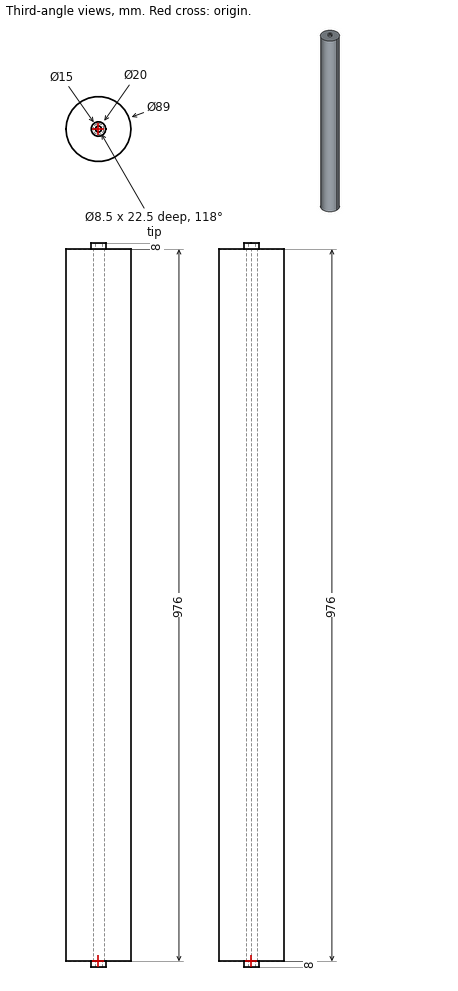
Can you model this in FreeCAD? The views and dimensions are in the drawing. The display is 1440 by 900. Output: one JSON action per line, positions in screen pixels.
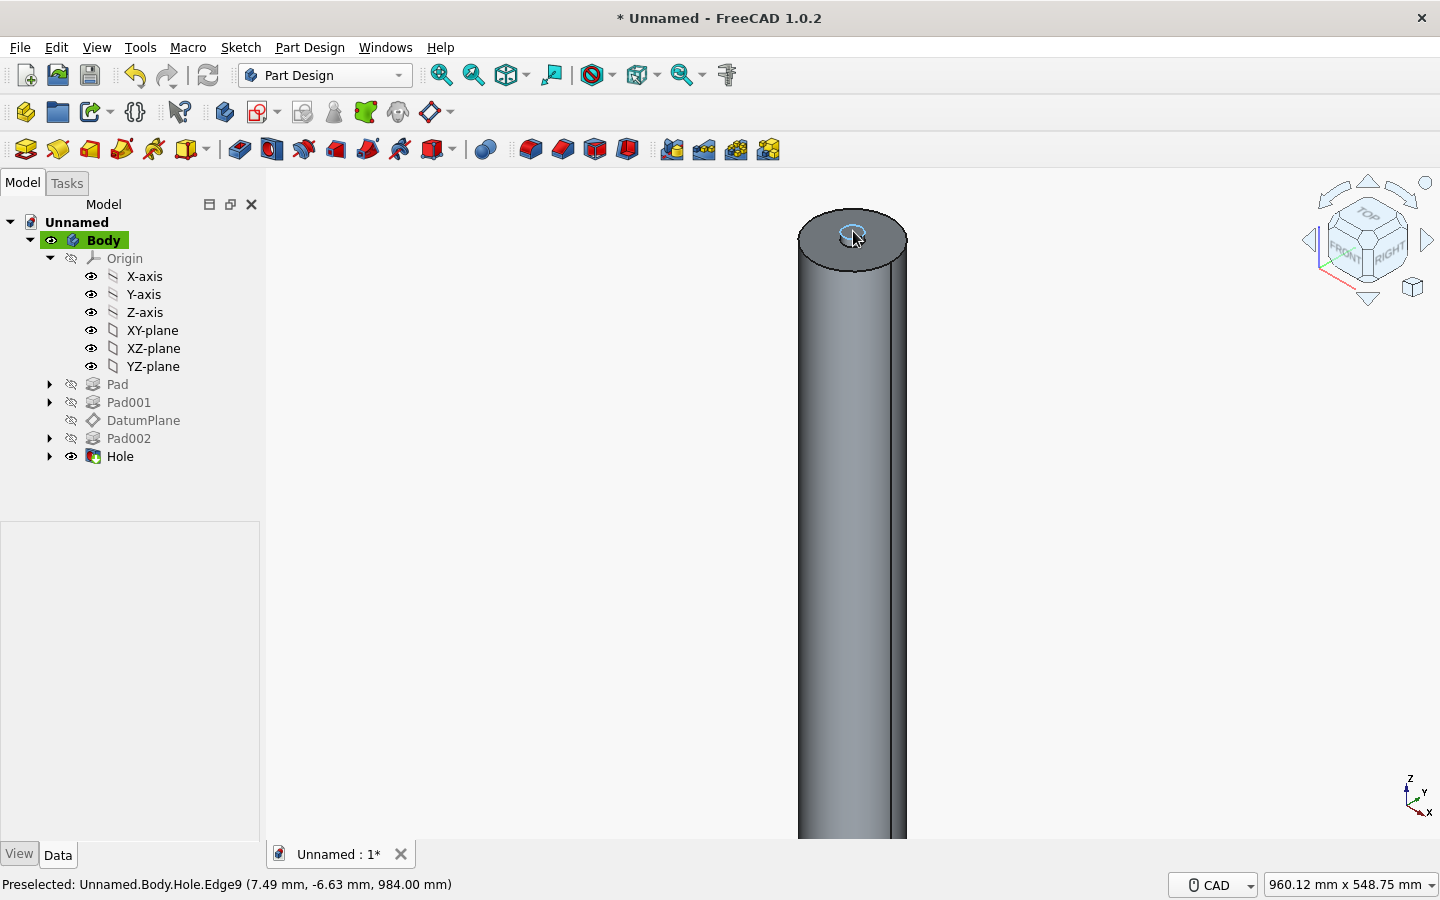
{"action": "left_click", "coordinate": [442, 76]}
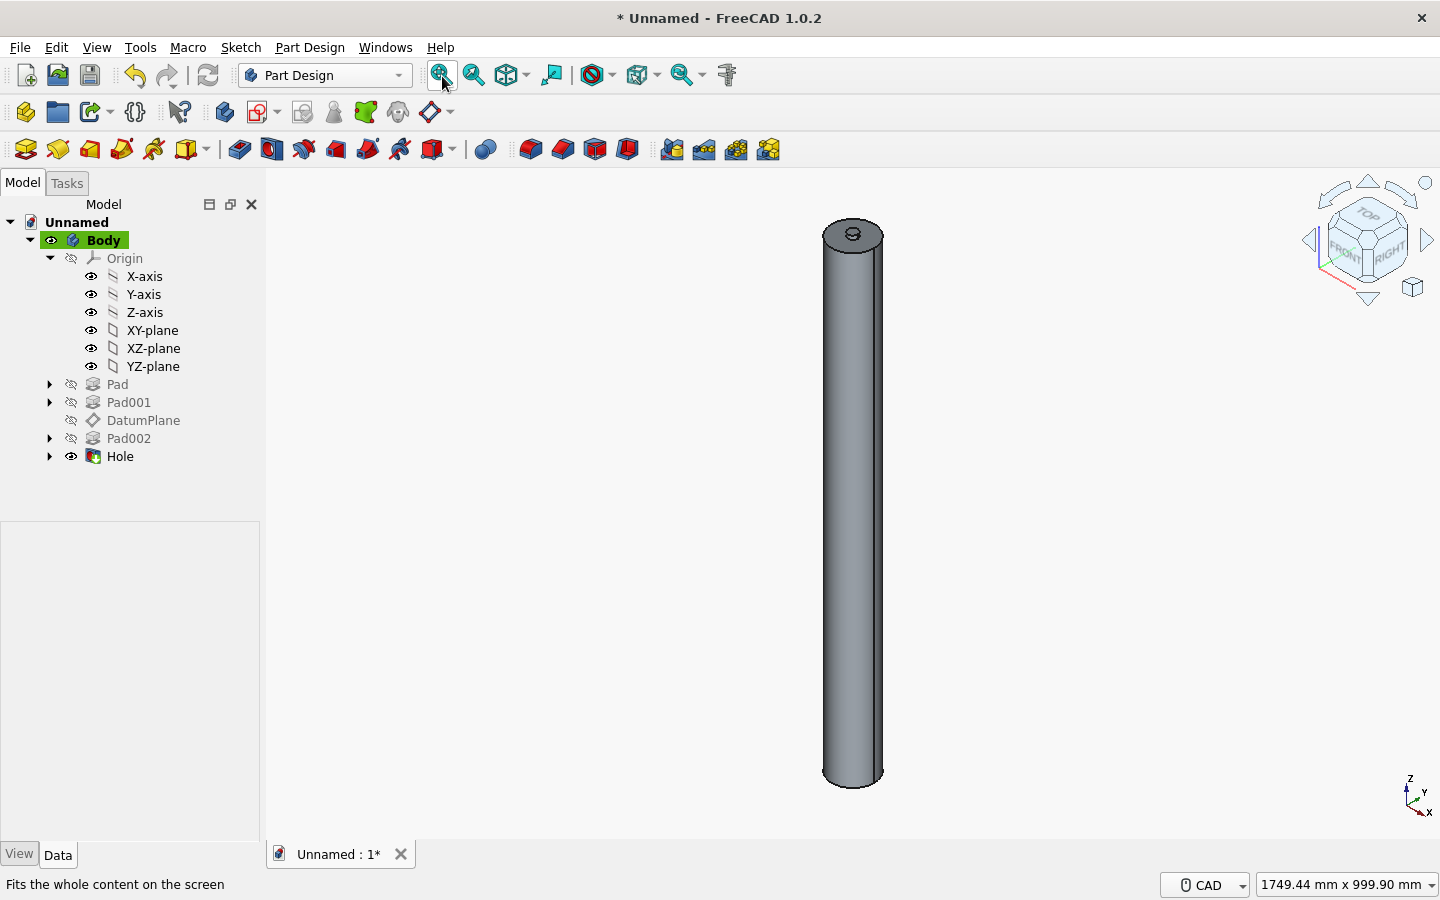
{"action": "key", "text": "2"}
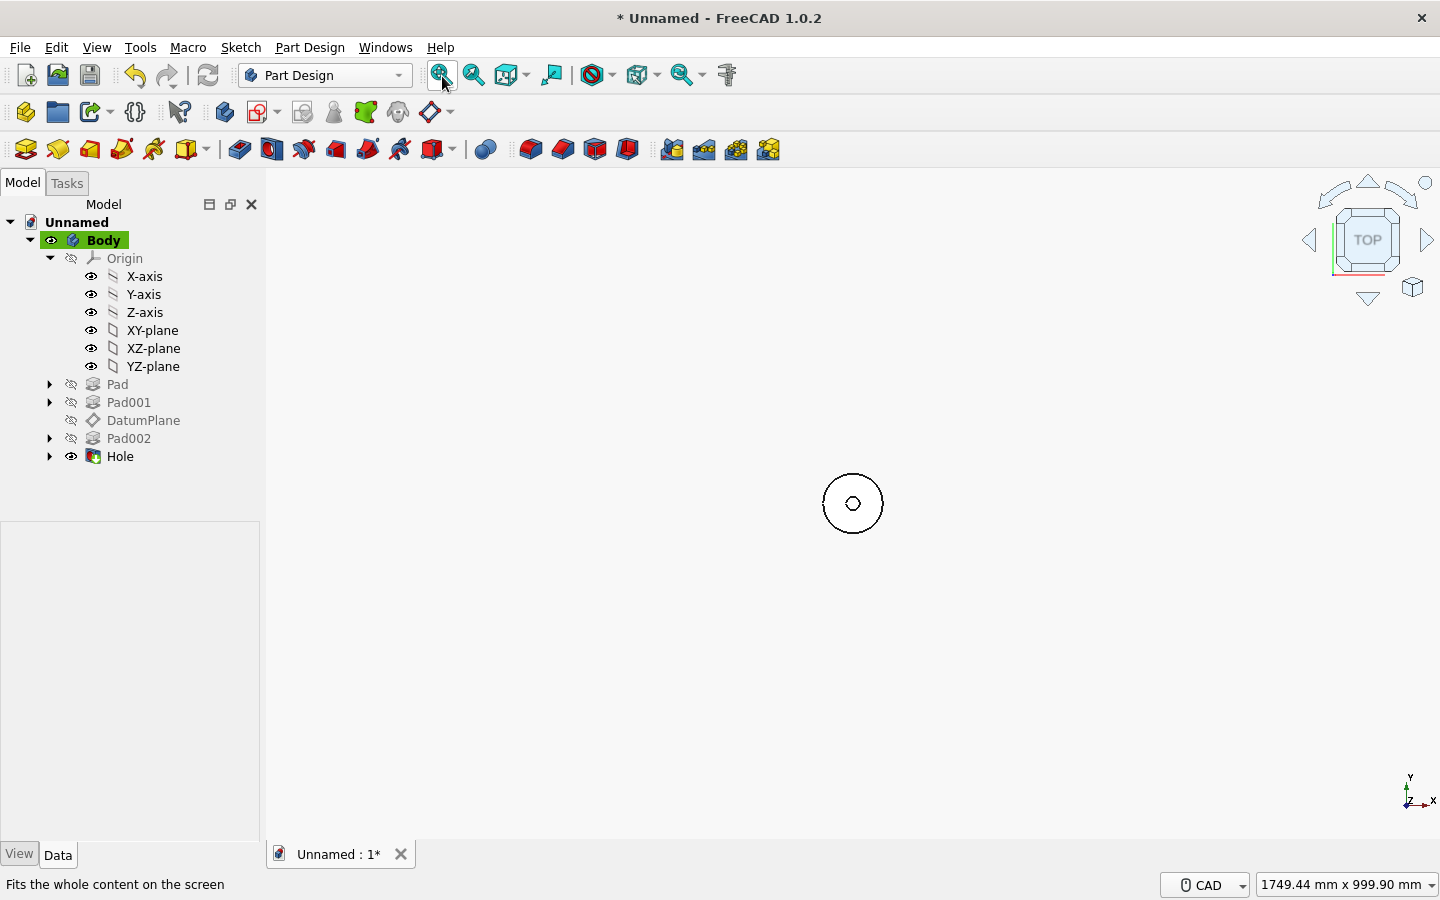
{"action": "left_click", "coordinate": [442, 76]}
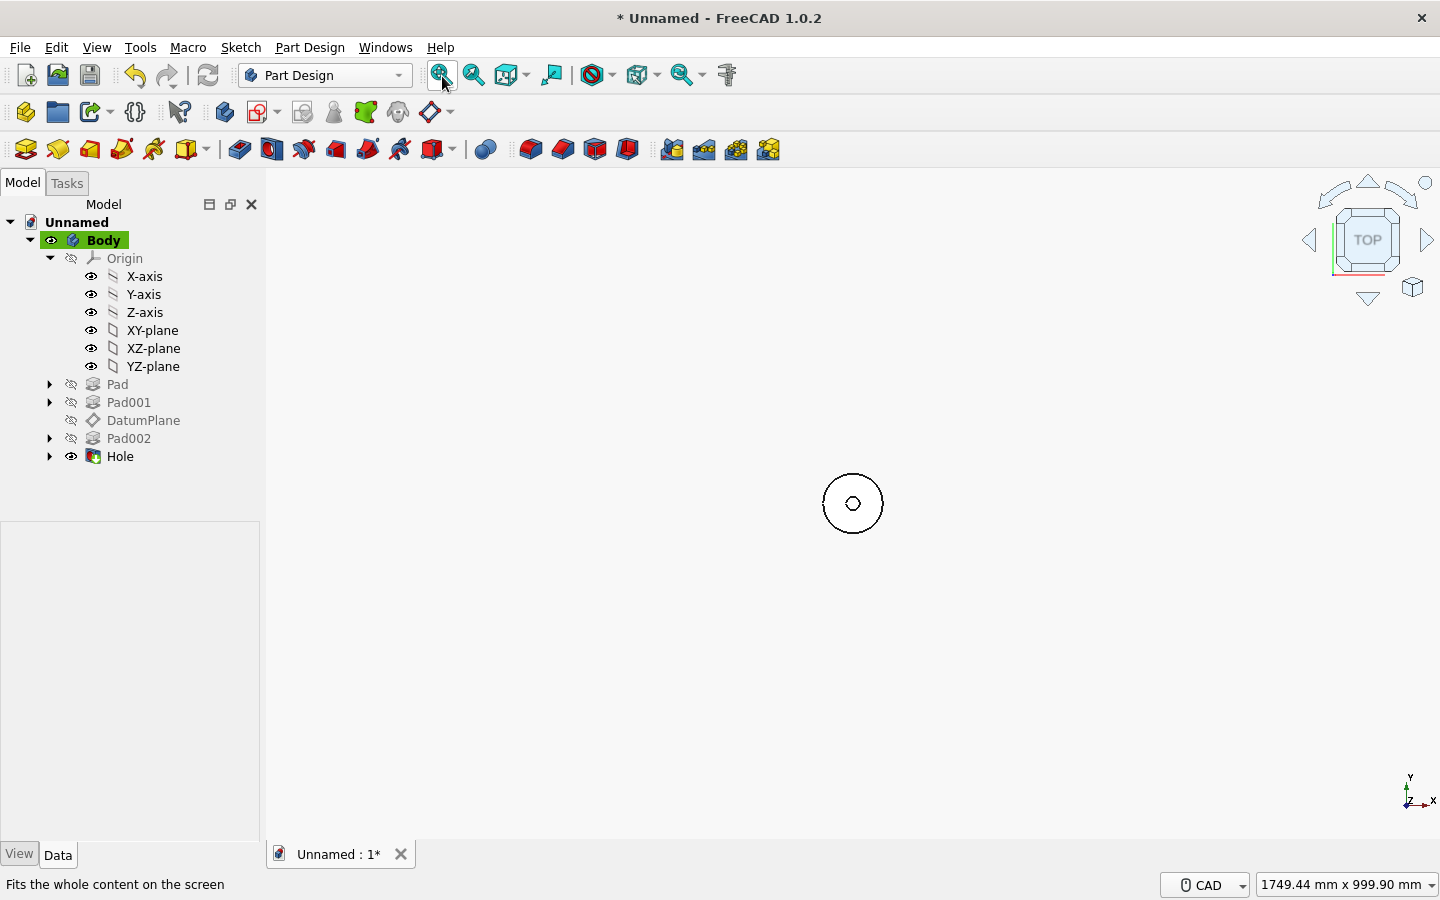
{"action": "scroll", "coordinate": [853, 502], "scroll_direction": "up", "scroll_amount": 3}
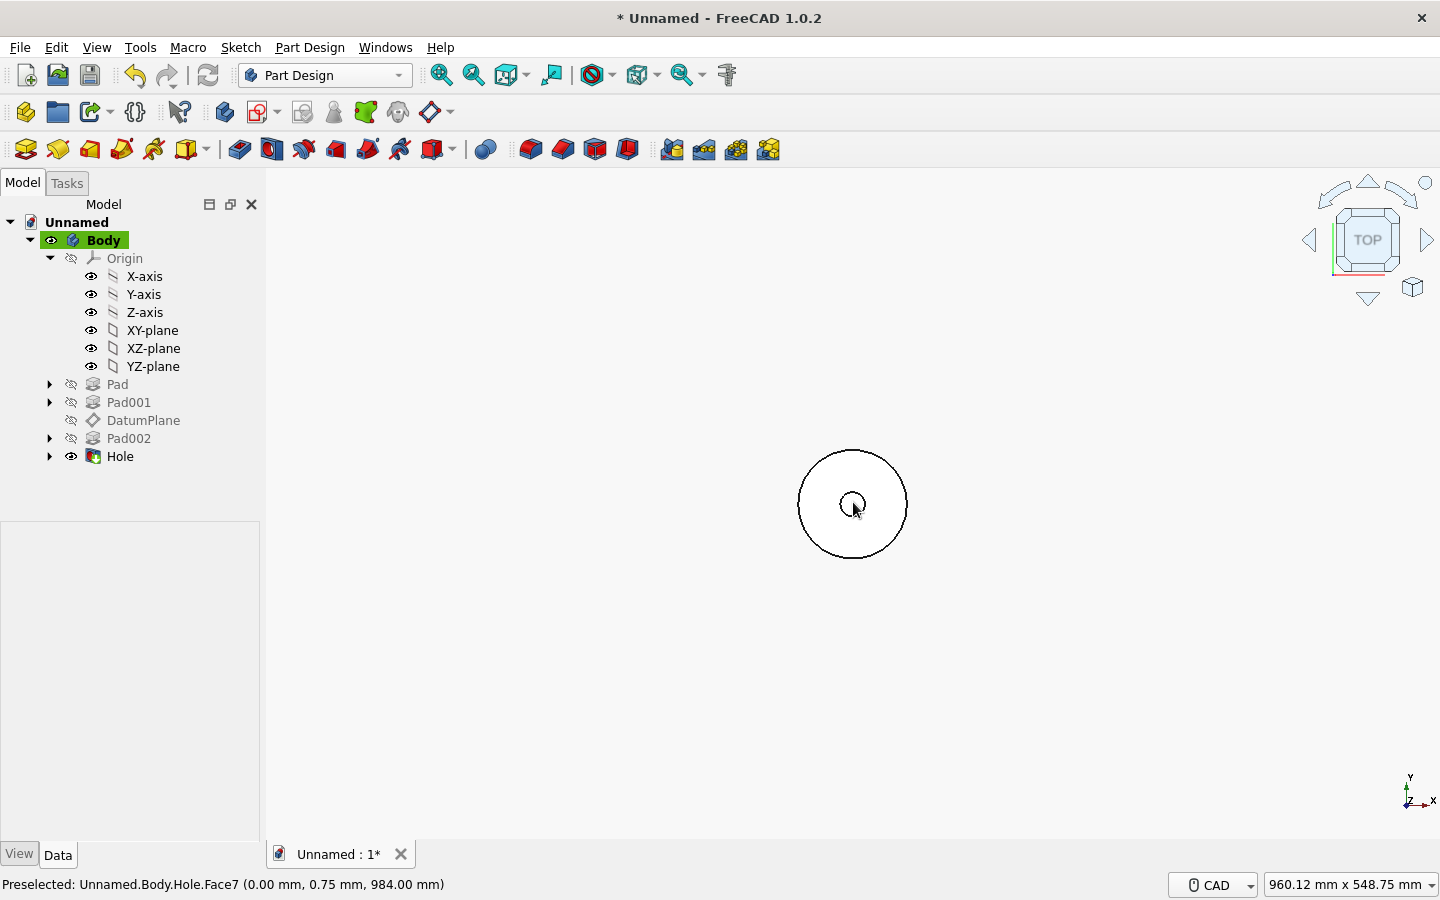
{"action": "left_click", "coordinate": [853, 503]}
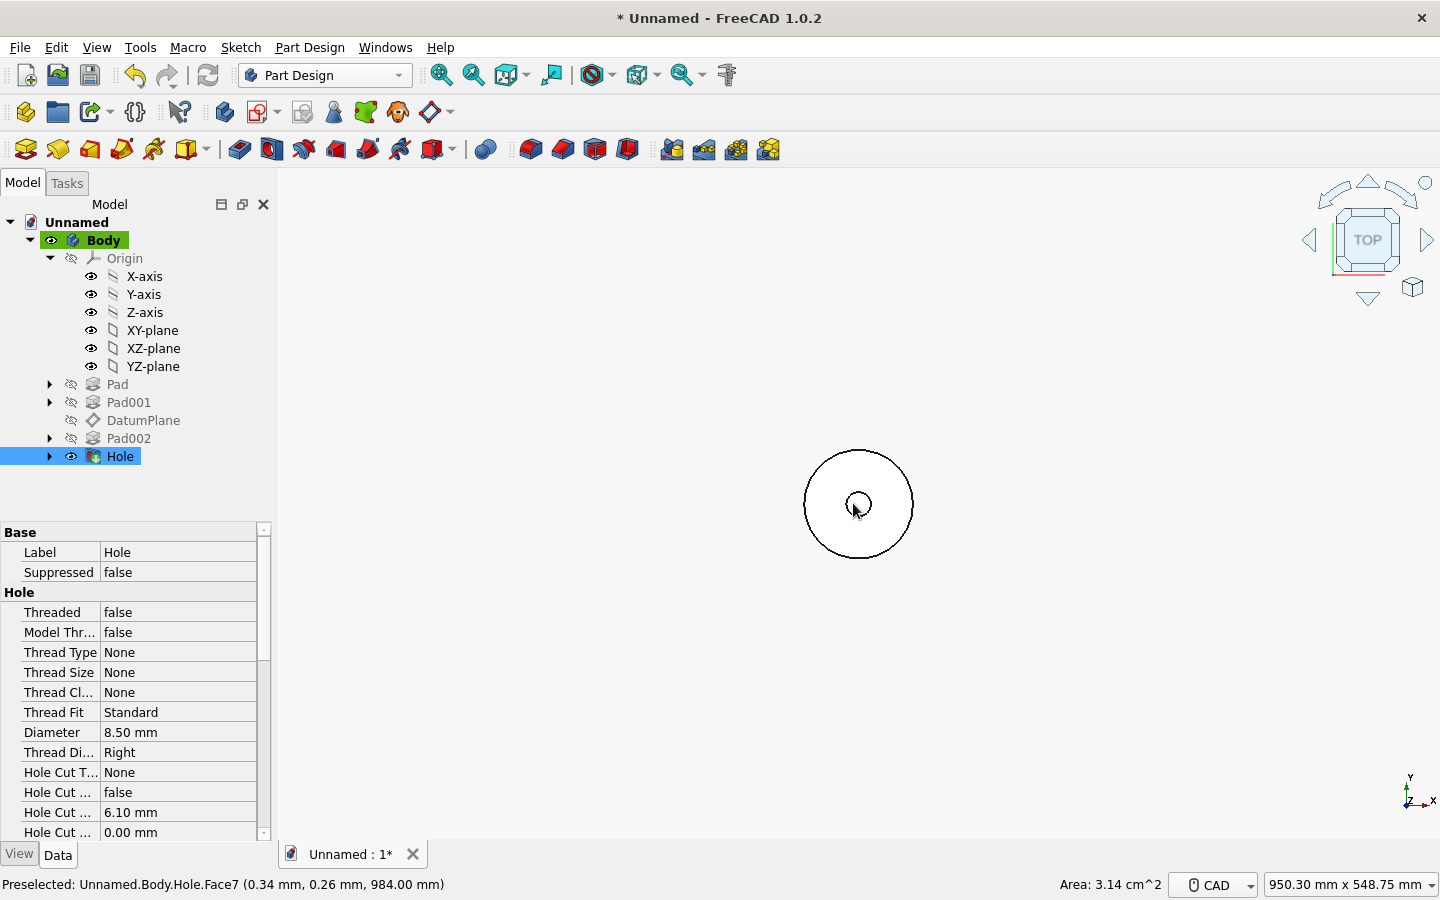
{"action": "left_click", "coordinate": [258, 112]}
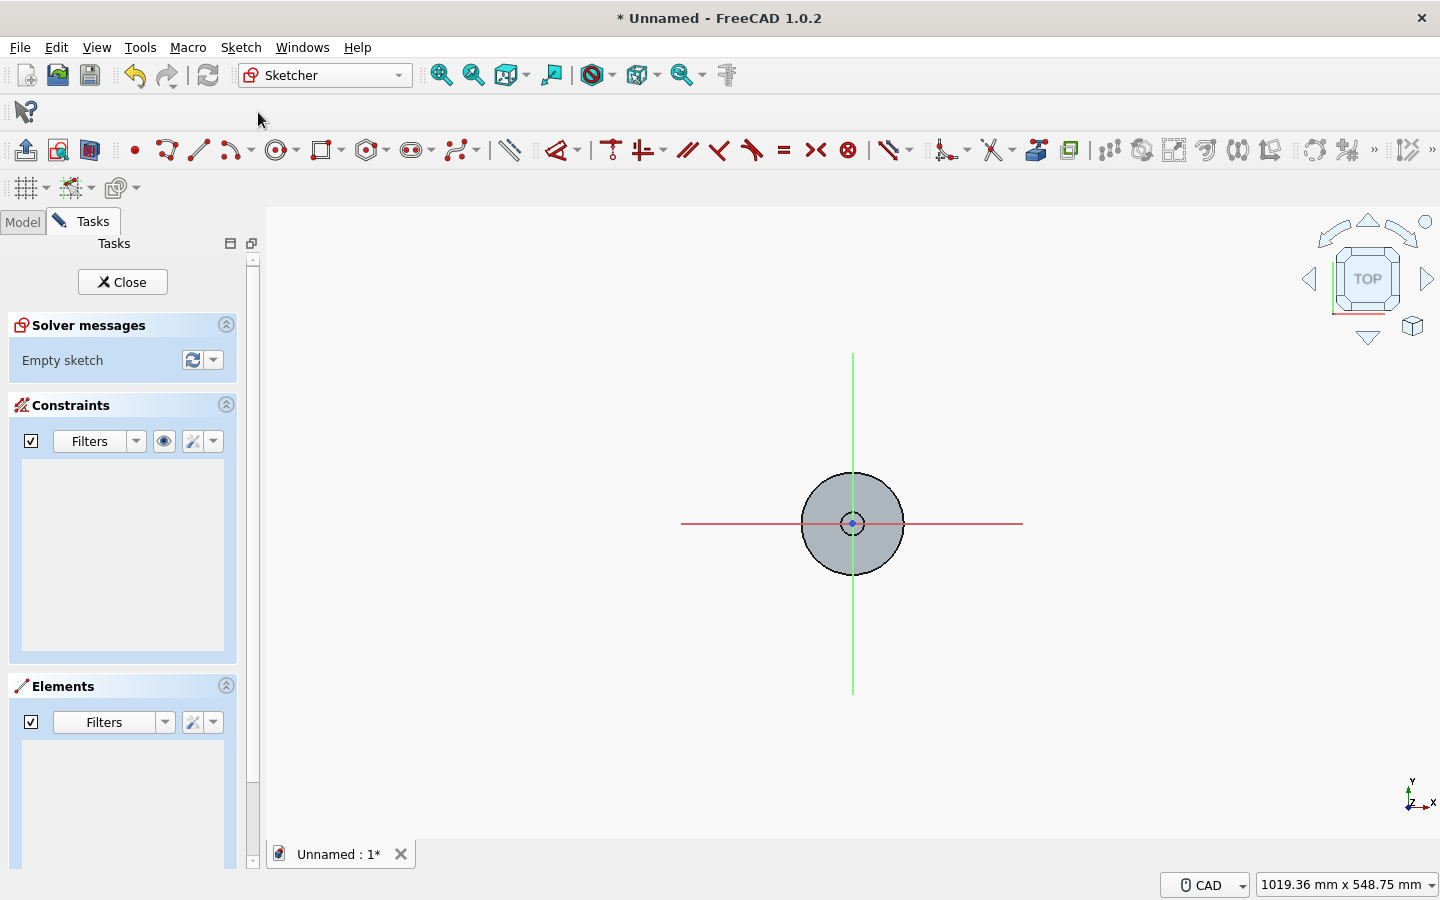
{"action": "scroll", "coordinate": [856, 524], "scroll_direction": "up", "scroll_amount": 15}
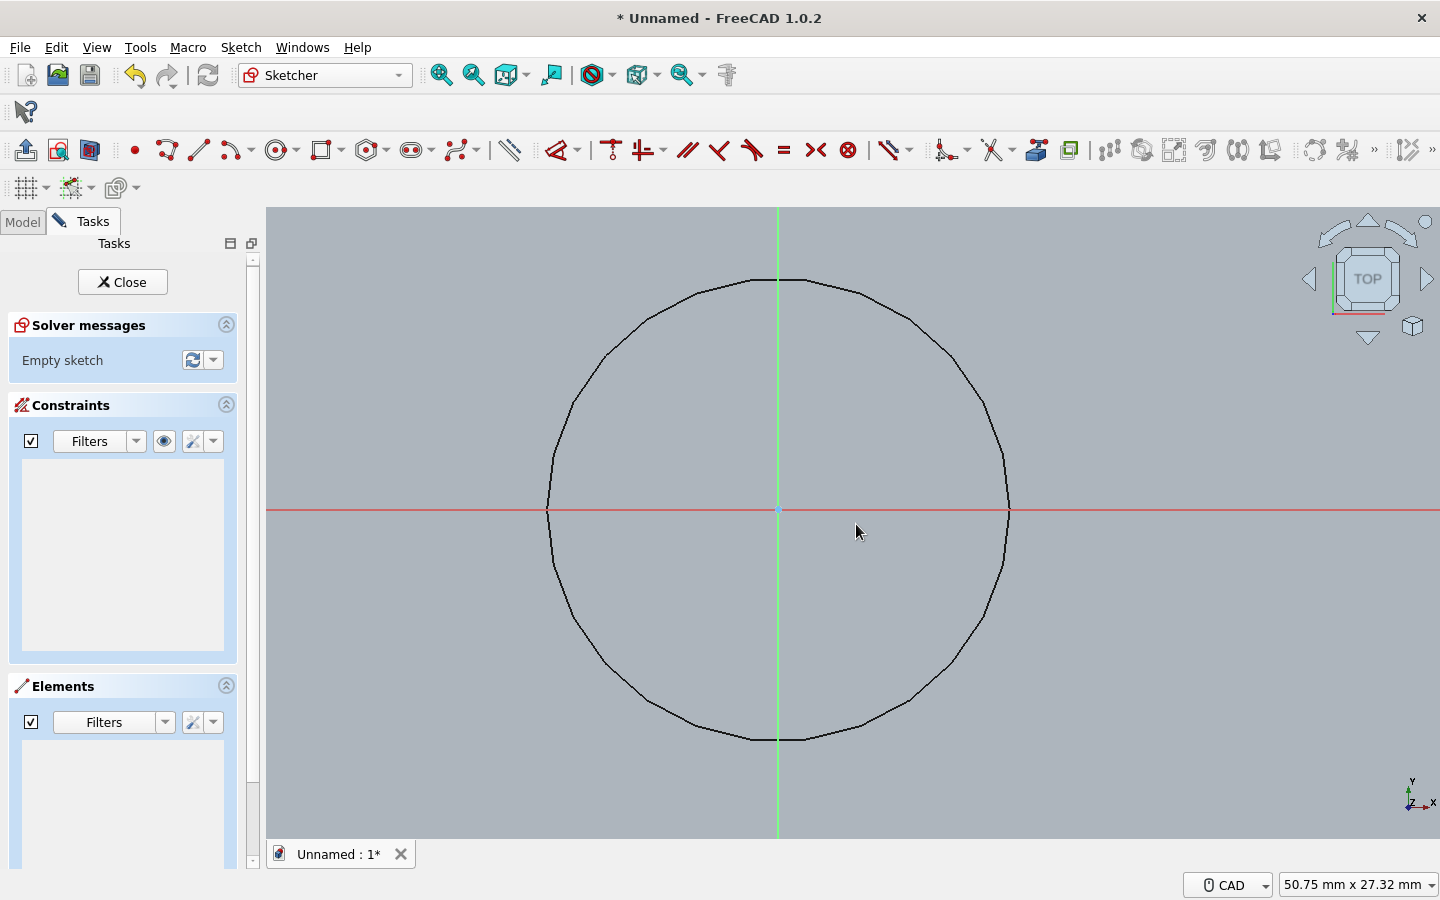
{"action": "scroll", "coordinate": [773, 499], "scroll_direction": "up", "scroll_amount": 4}